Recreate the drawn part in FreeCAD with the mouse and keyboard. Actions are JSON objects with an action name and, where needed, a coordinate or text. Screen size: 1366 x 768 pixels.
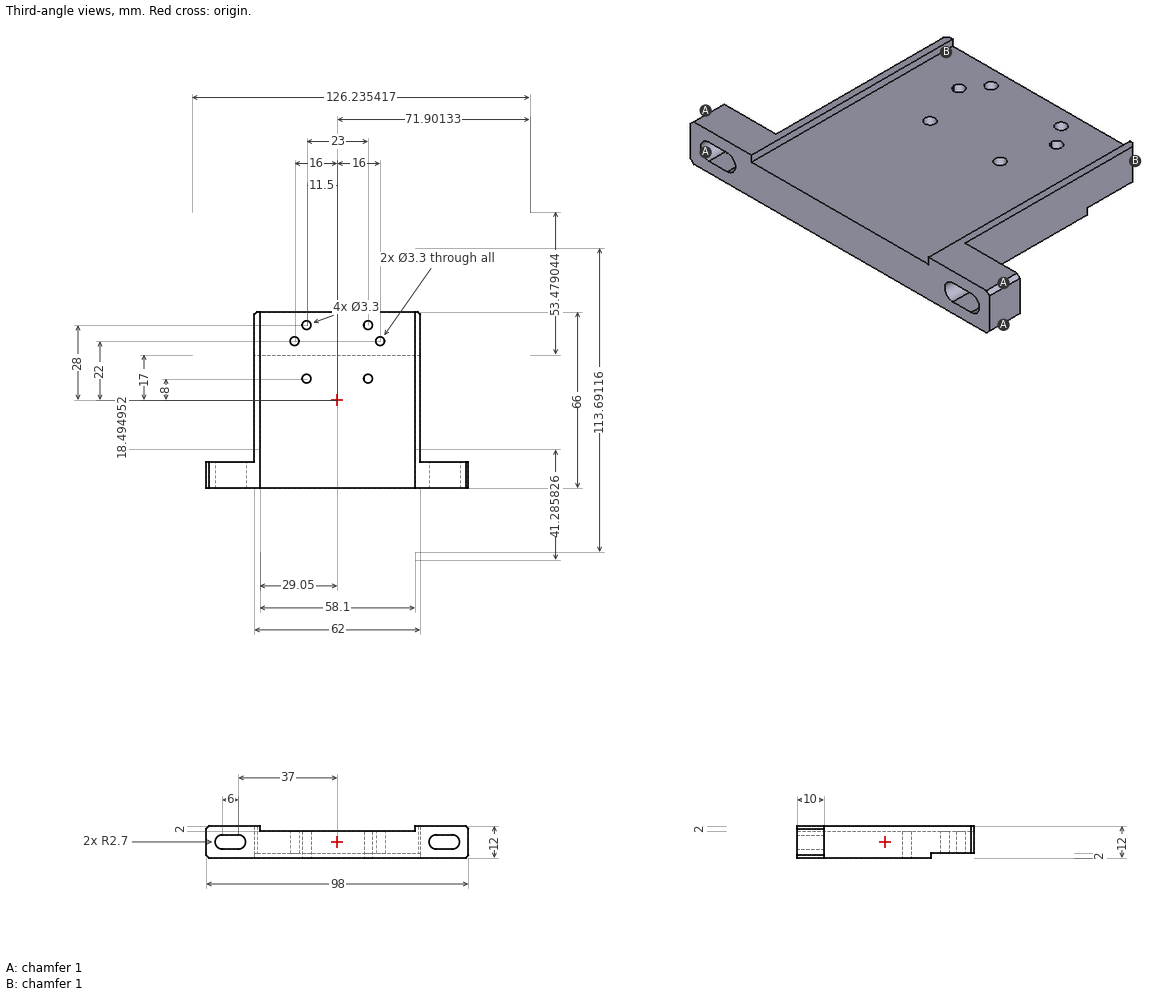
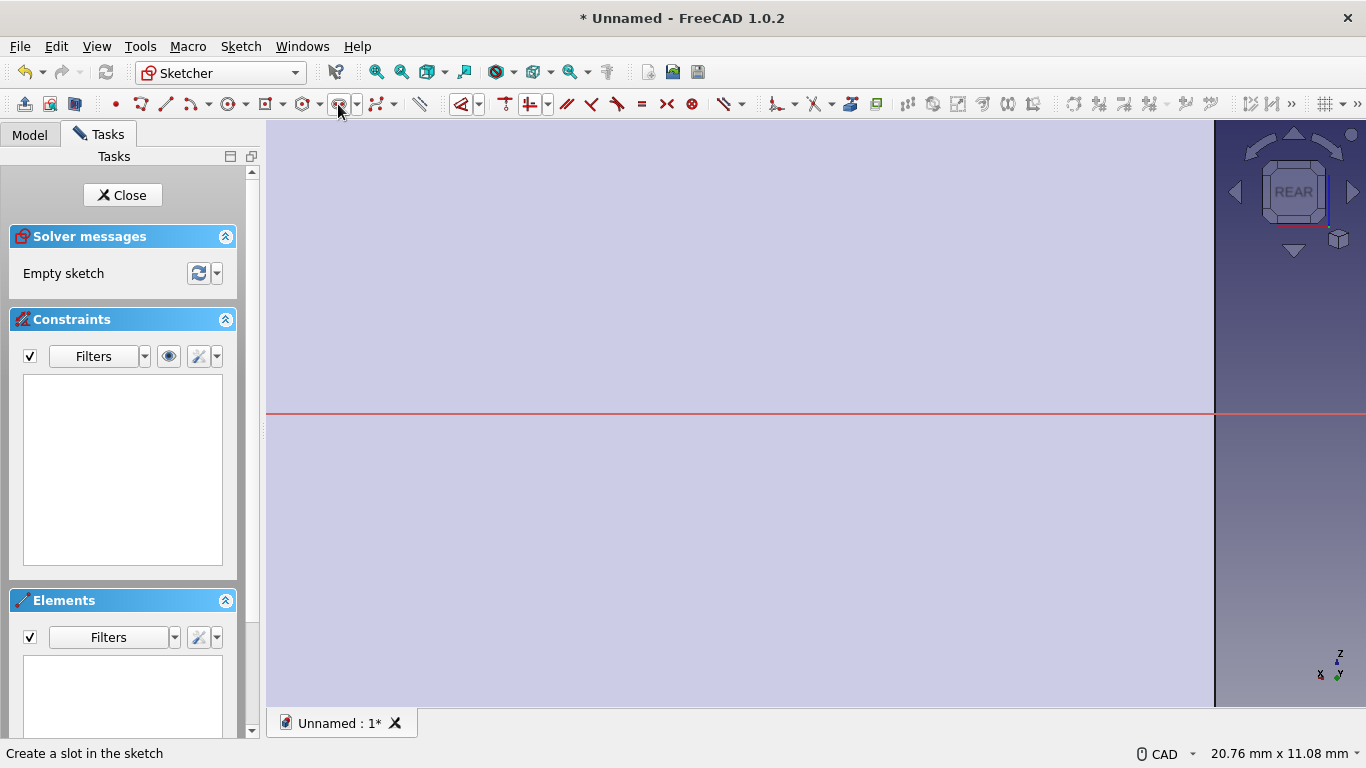
{"action": "left_click", "coordinate": [579, 413]}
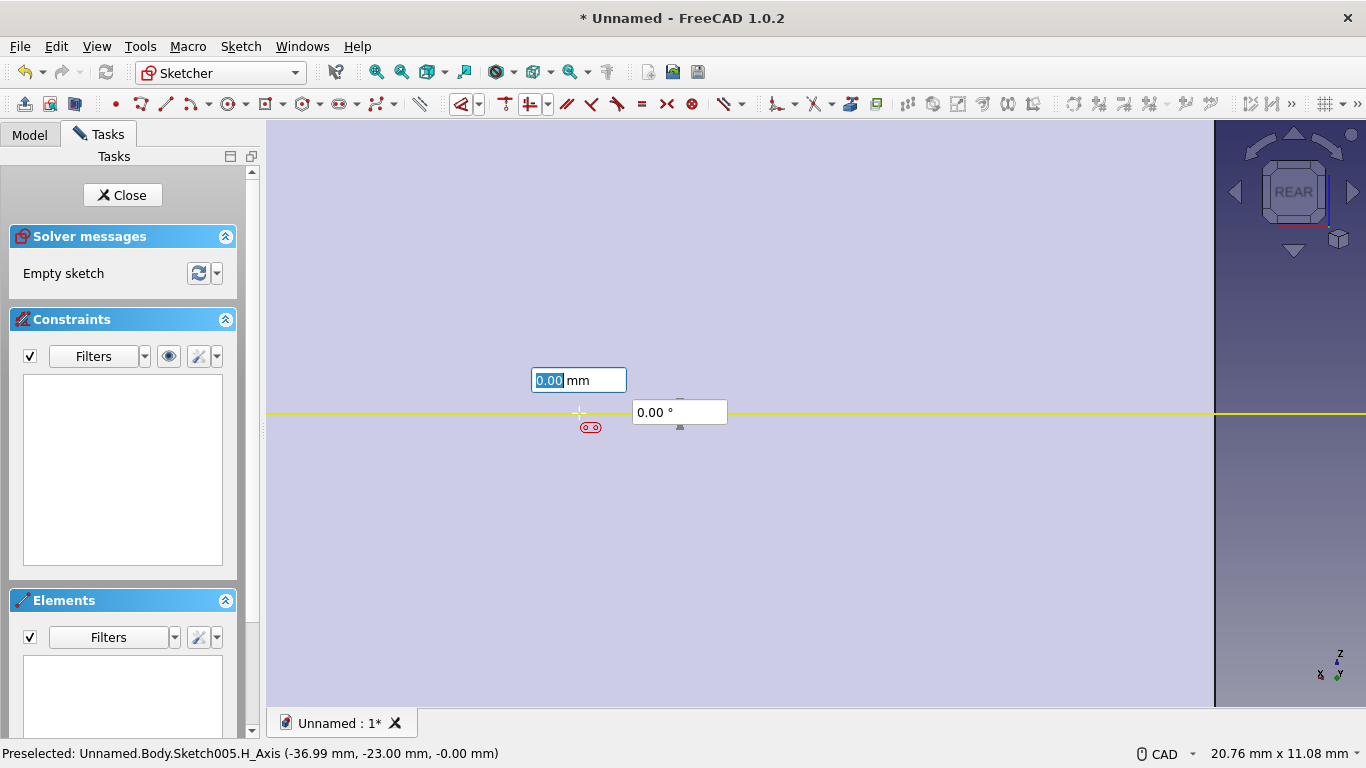
{"action": "left_click", "coordinate": [897, 404]}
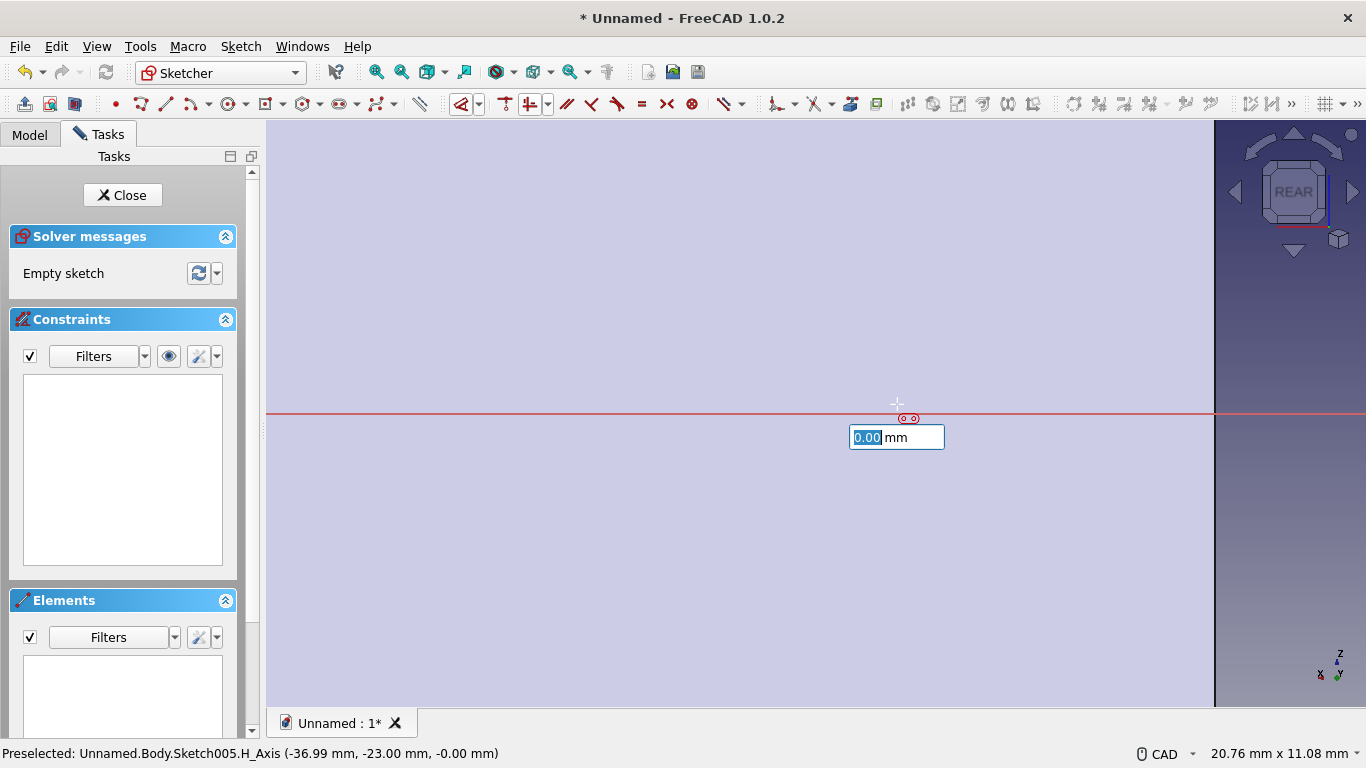
{"action": "left_click", "coordinate": [738, 557]}
{"action": "key", "text": "Escape"}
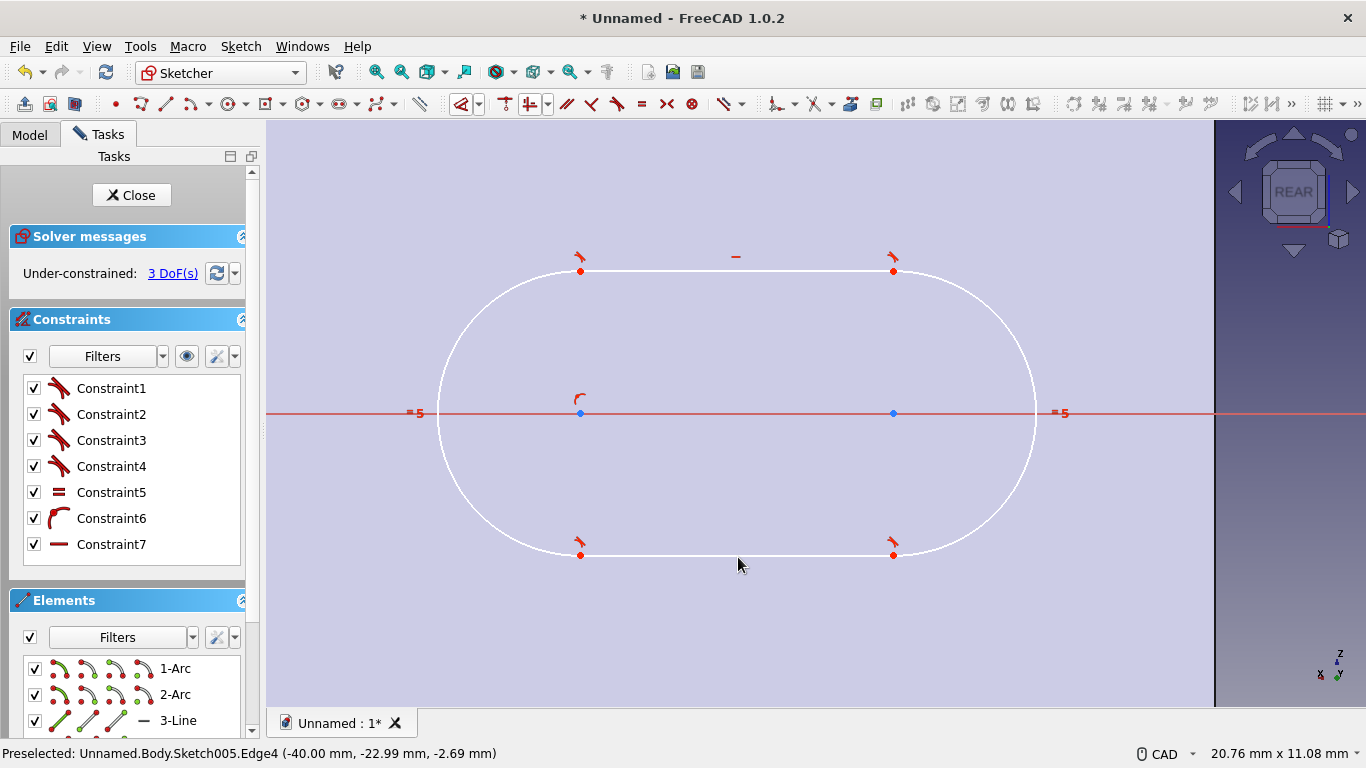
{"action": "left_click", "coordinate": [465, 330]}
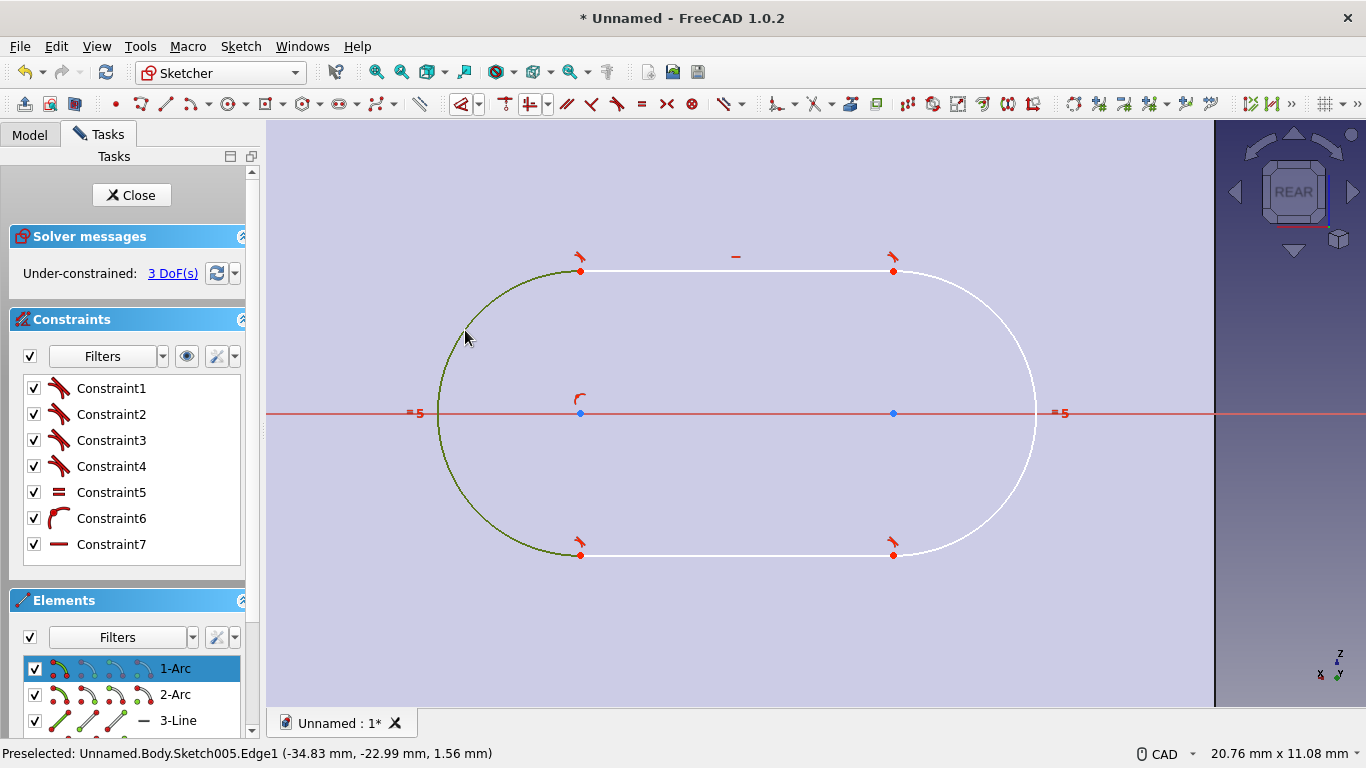
{"action": "key", "text": "k r"}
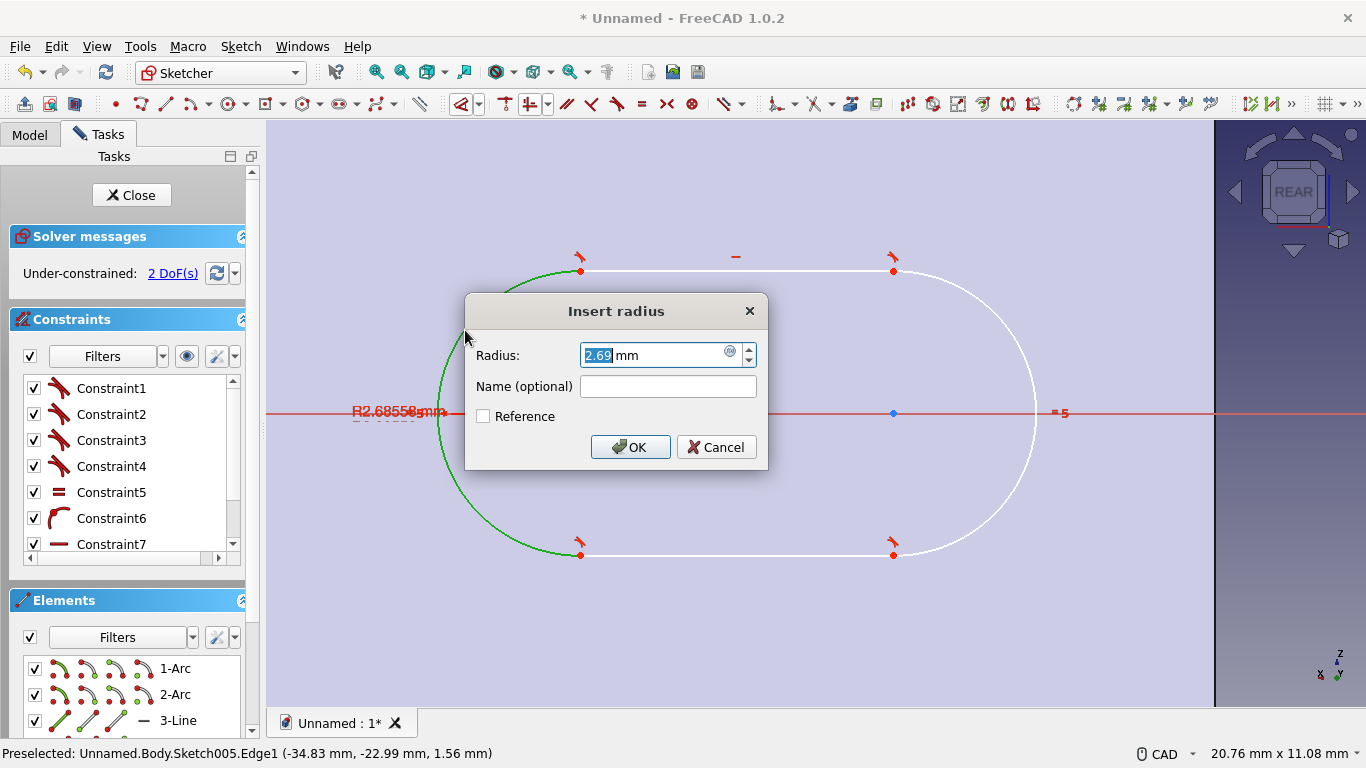
{"action": "type", "text": "2.7"}
{"action": "key", "text": "Return"}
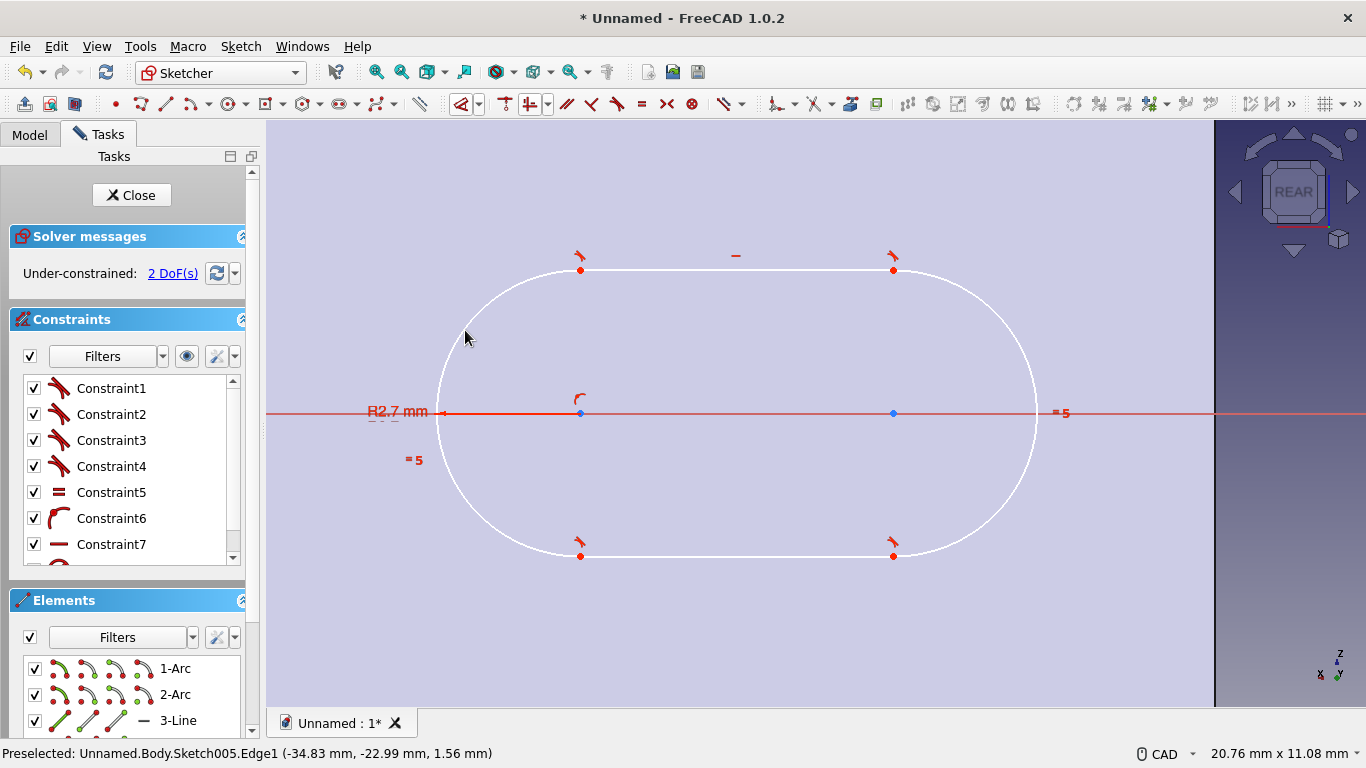
{"action": "left_click", "coordinate": [674, 270]}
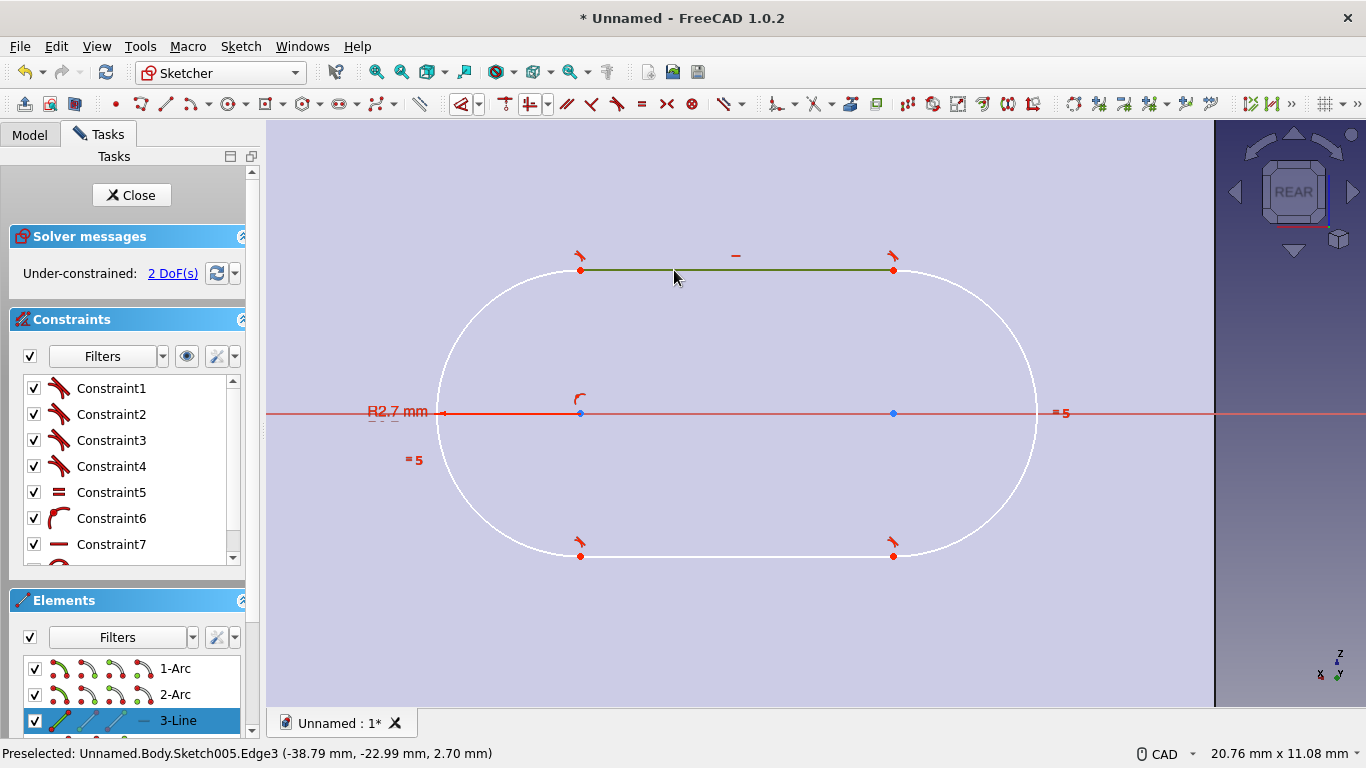
{"action": "left_click", "coordinate": [478, 104]}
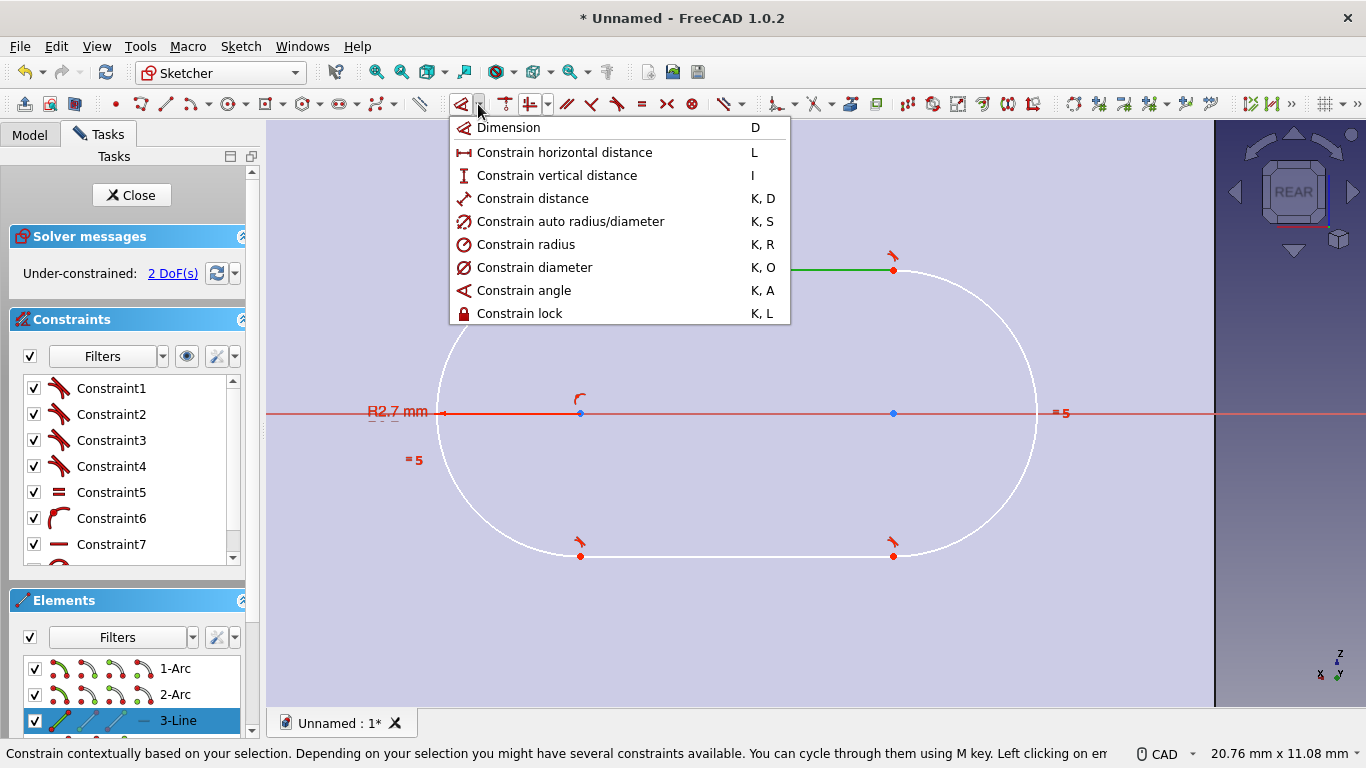
{"action": "left_click", "coordinate": [620, 152]}